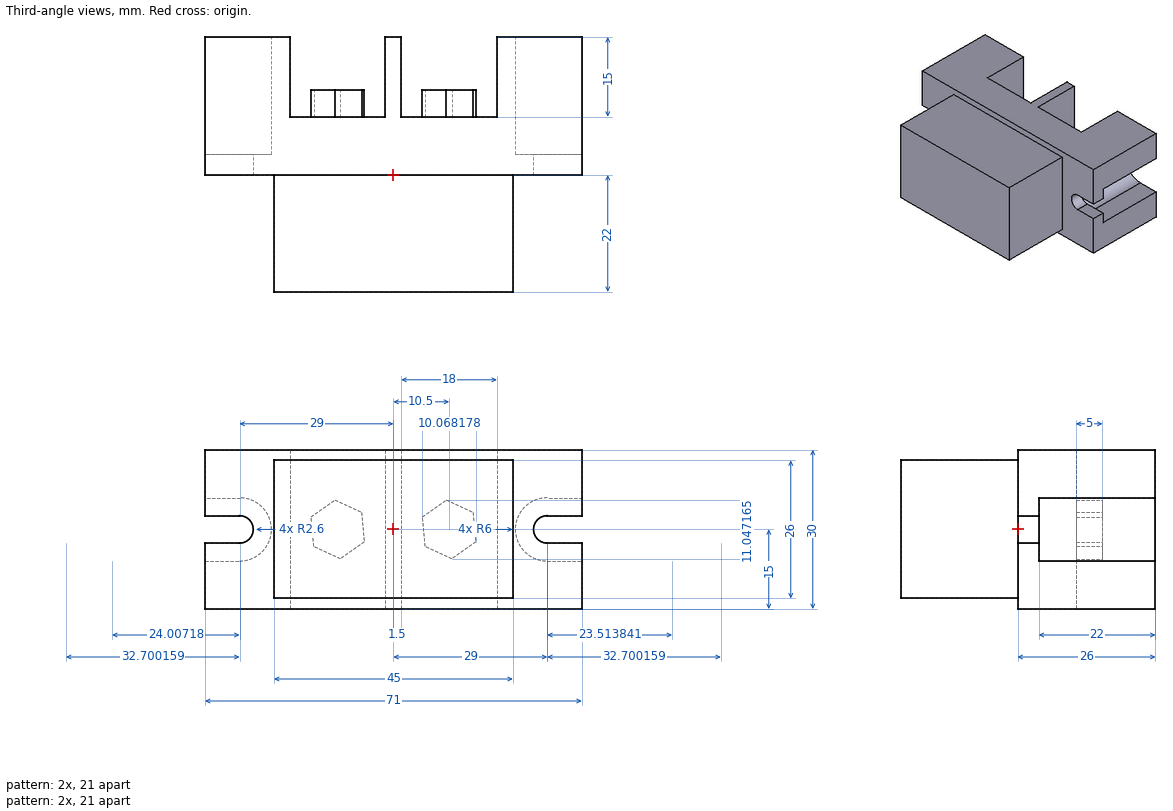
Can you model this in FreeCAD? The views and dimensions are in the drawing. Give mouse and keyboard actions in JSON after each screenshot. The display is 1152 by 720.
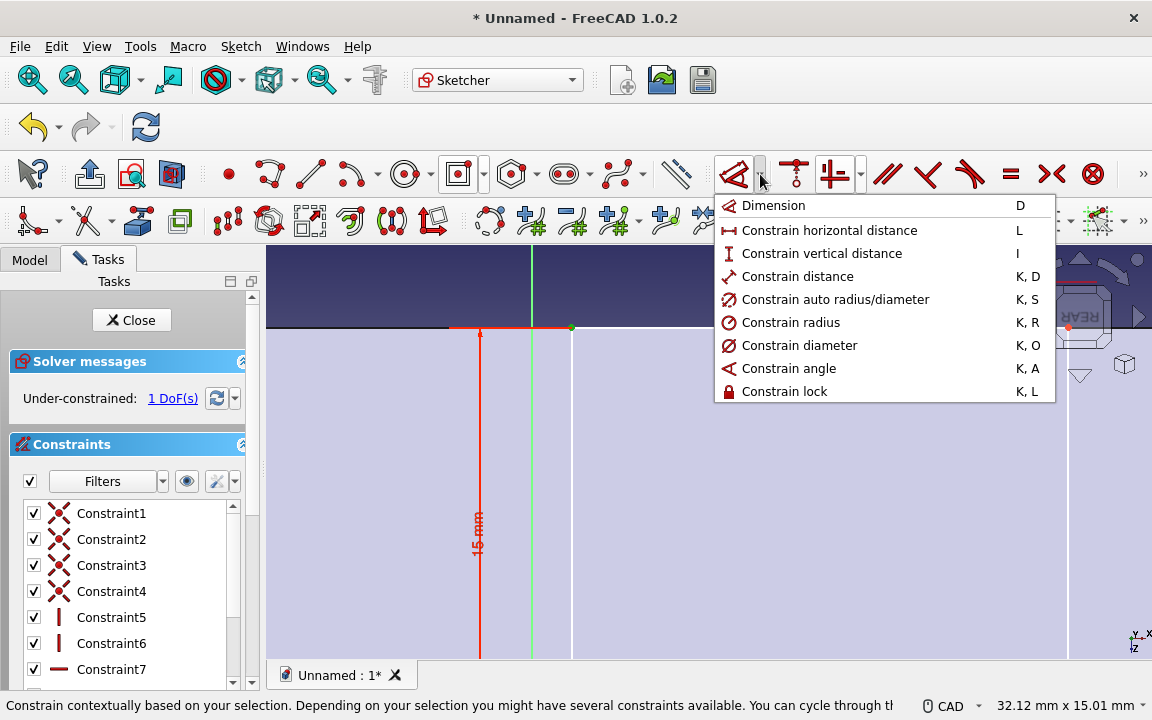
{"action": "left_click", "coordinate": [885, 230]}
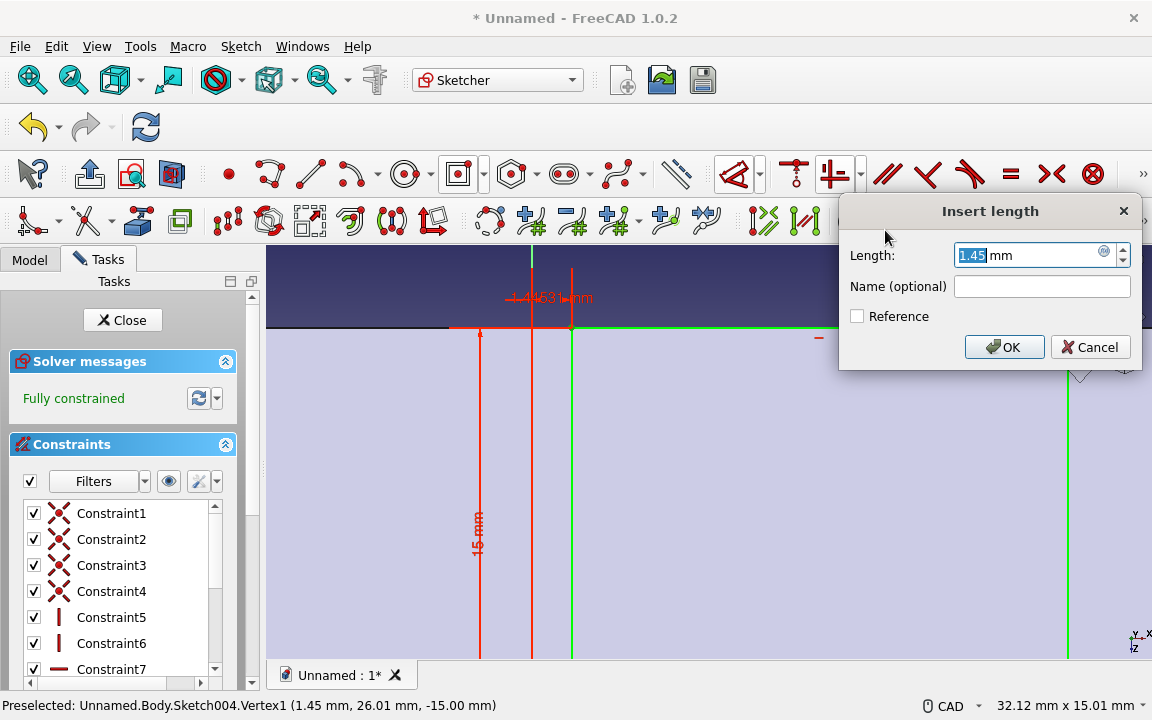
{"action": "type", "text": "1.5"}
{"action": "key", "text": "Return"}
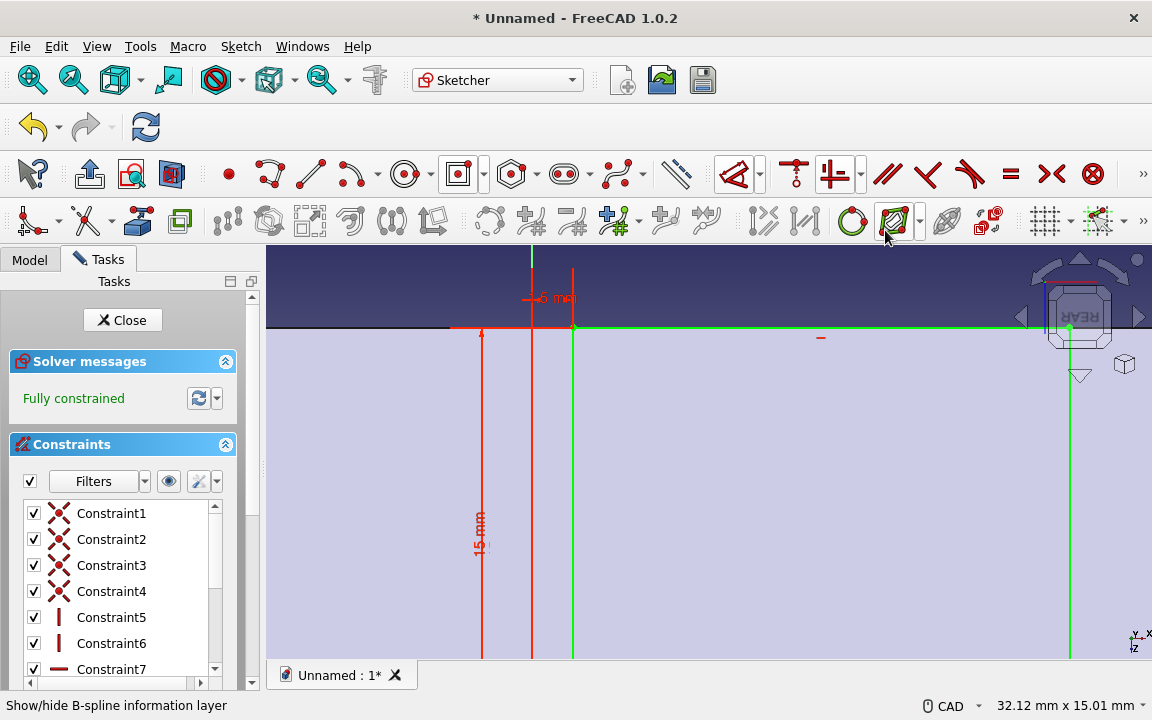
{"action": "left_click", "coordinate": [123, 320]}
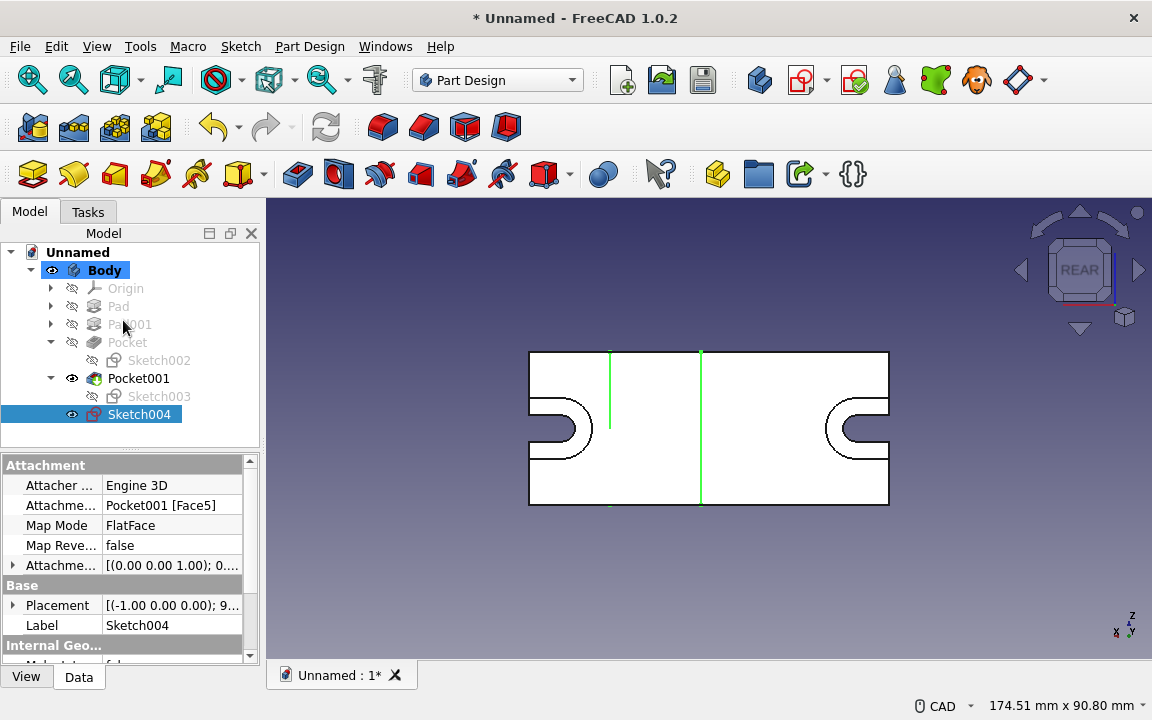
{"action": "left_click", "coordinate": [298, 174]}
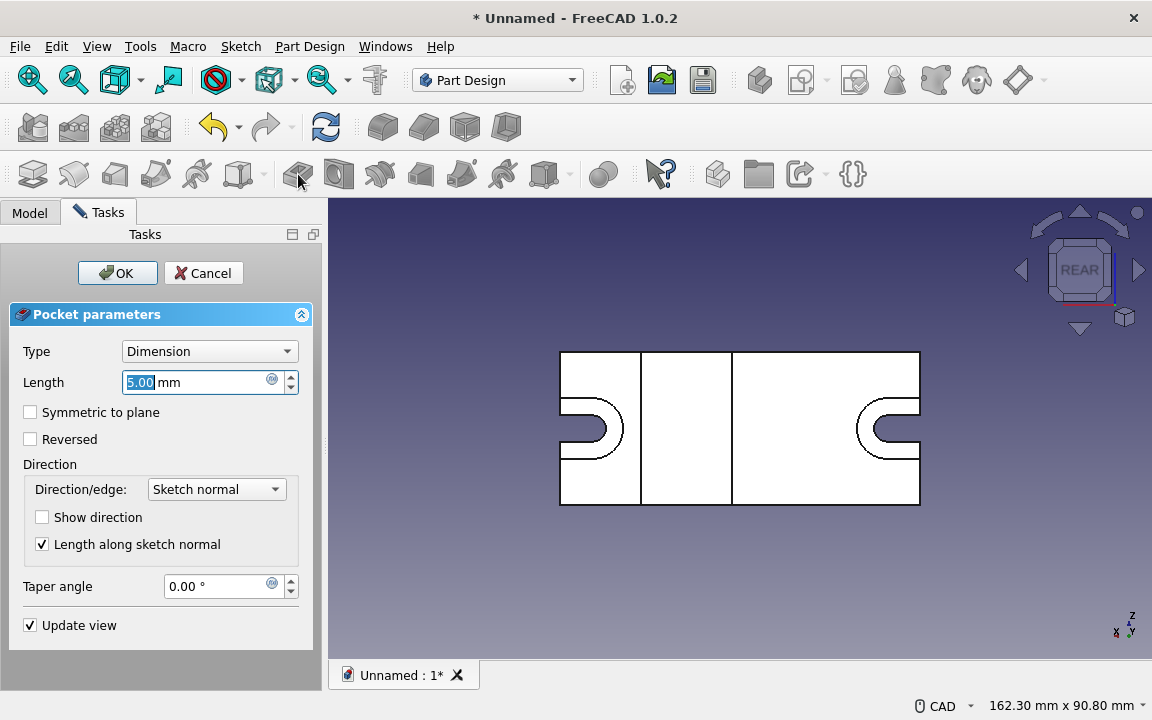
{"action": "type", "text": "15"}
{"action": "key", "text": "Tab"}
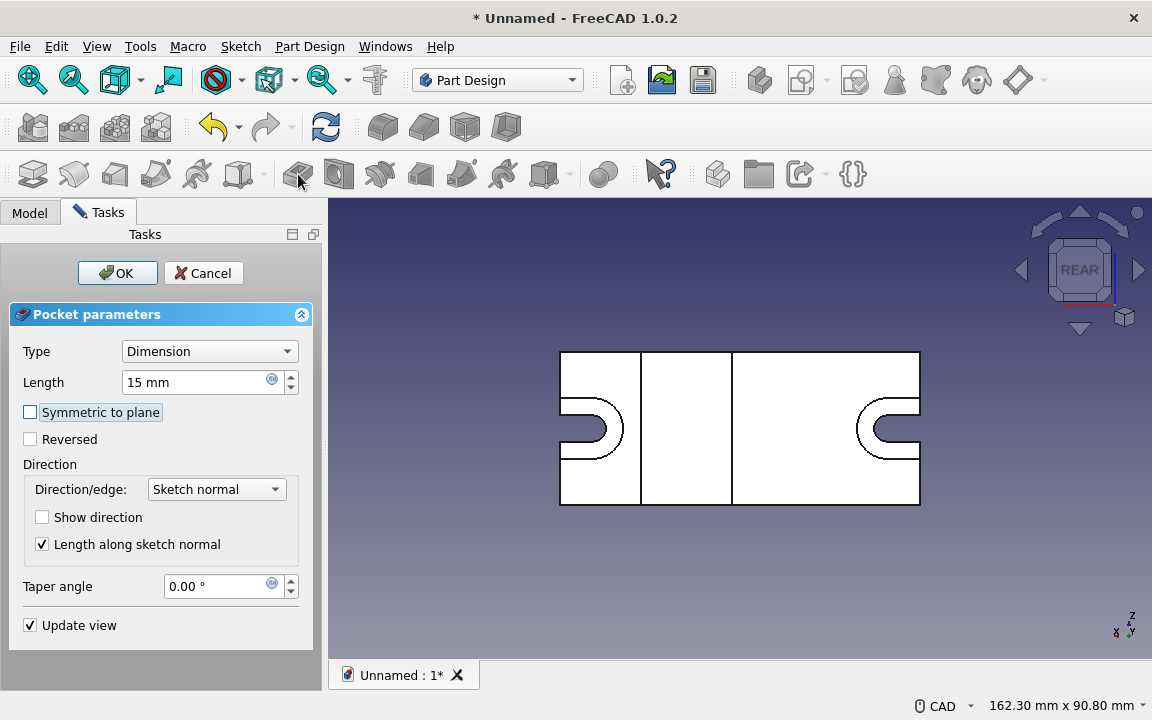
{"action": "left_click", "coordinate": [118, 273]}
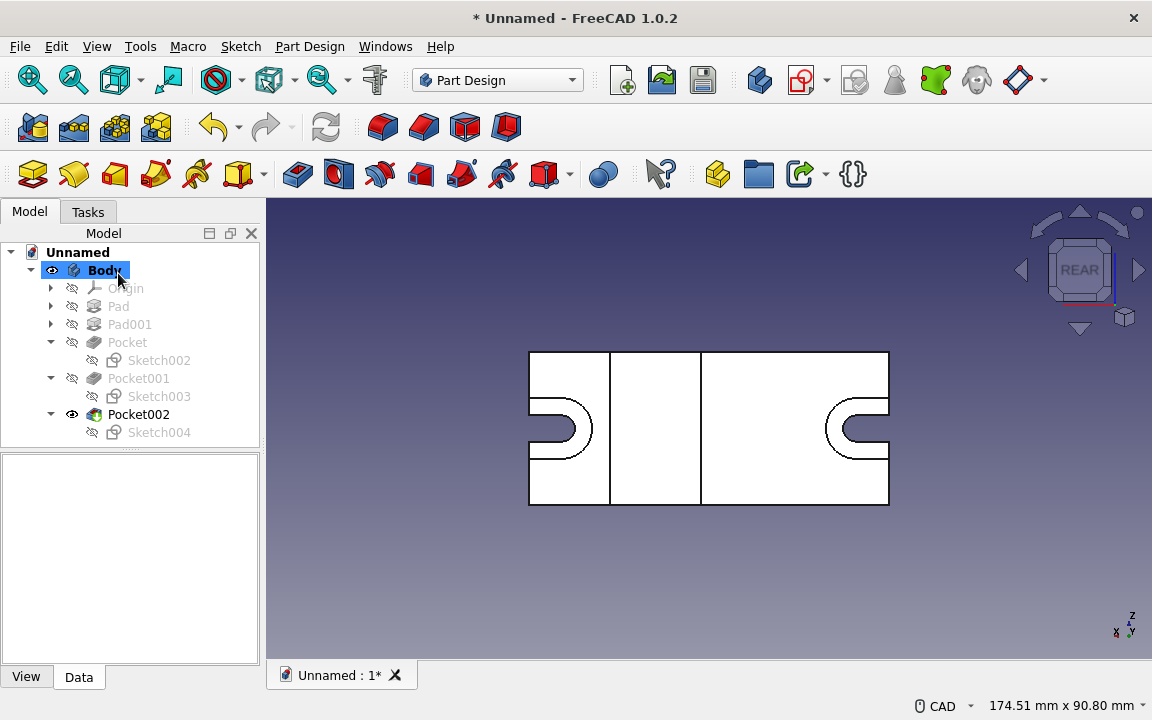
{"action": "left_click", "coordinate": [33, 80]}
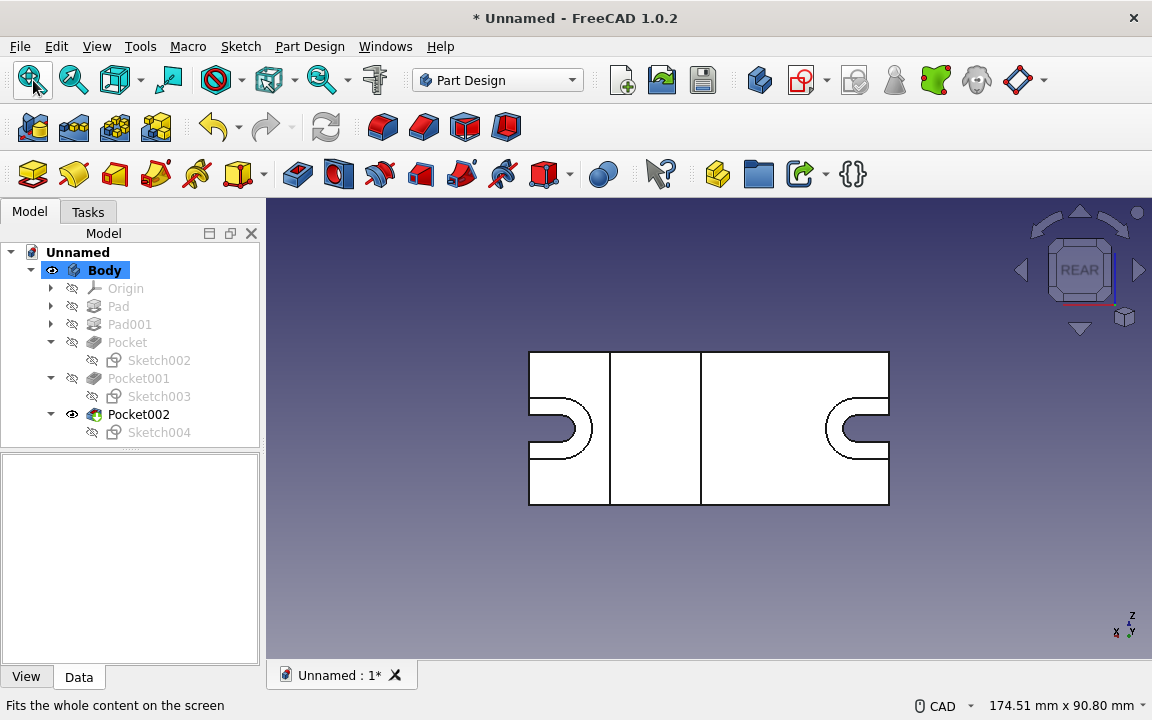
{"action": "left_click", "coordinate": [117, 414]}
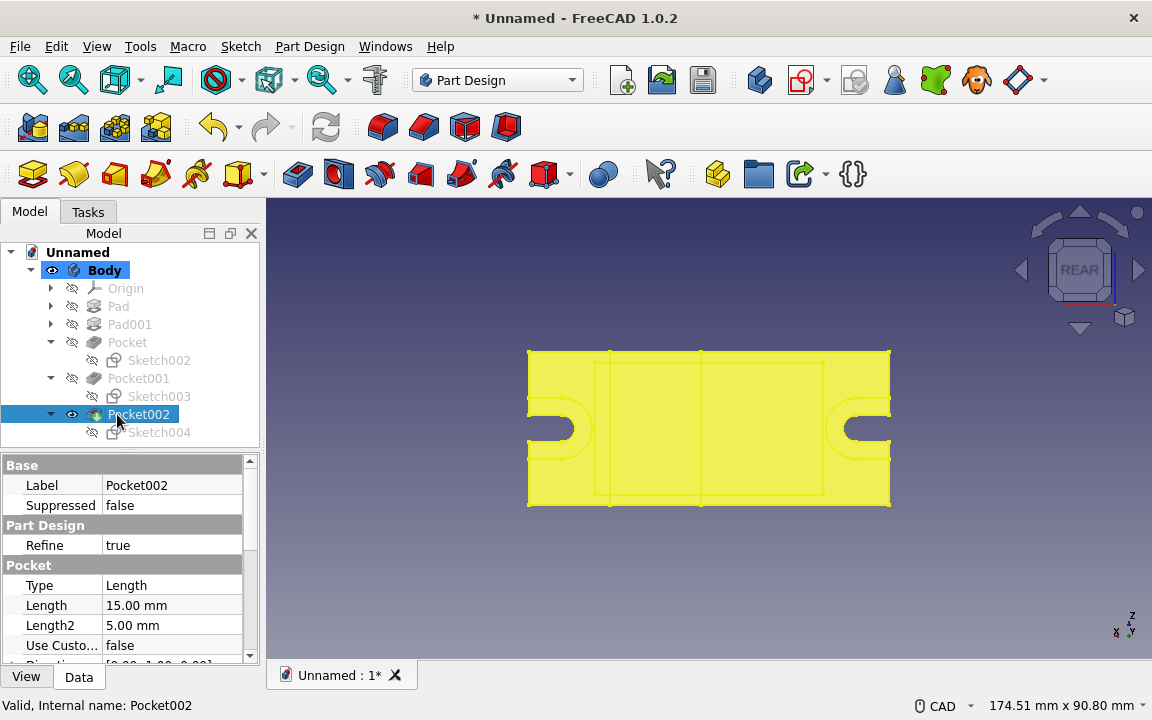
{"action": "left_click", "coordinate": [74, 128]}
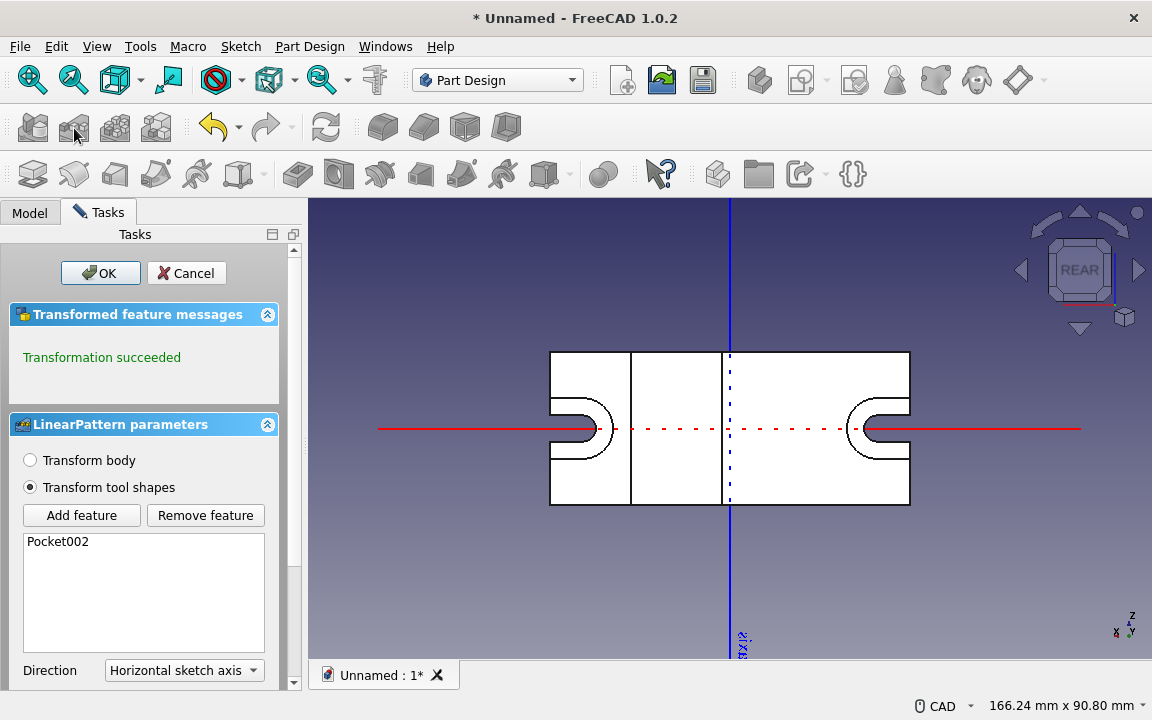
{"action": "left_click", "coordinate": [185, 670]}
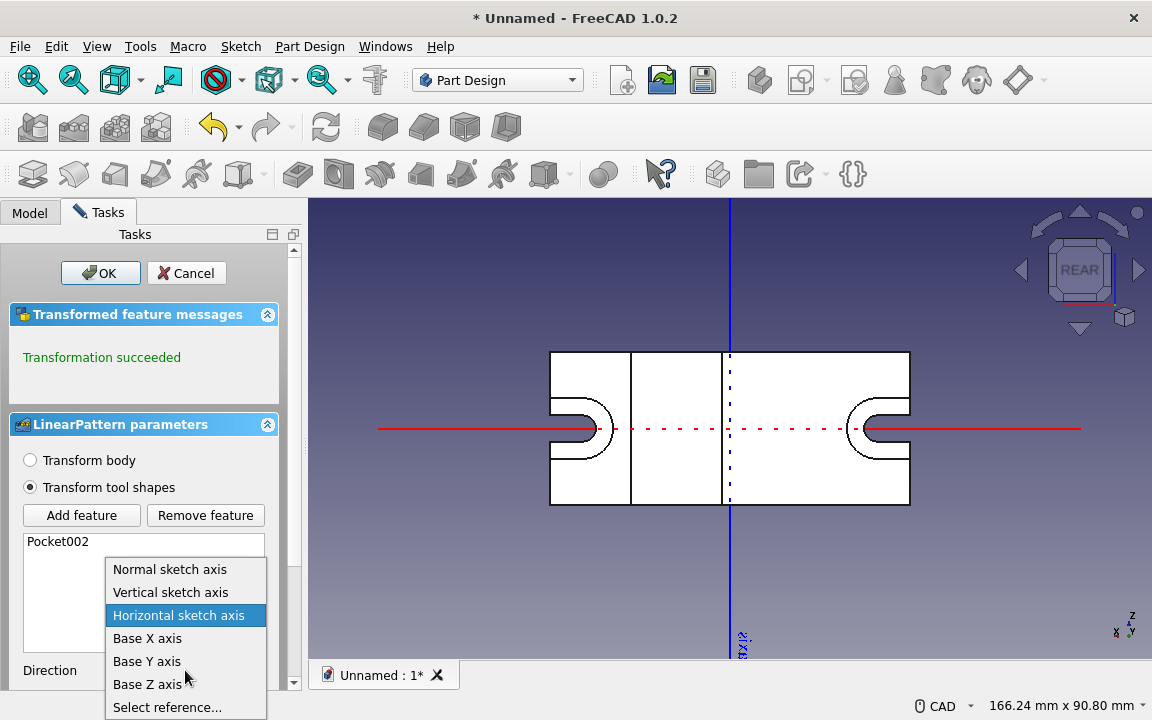
{"action": "left_click", "coordinate": [184, 638]}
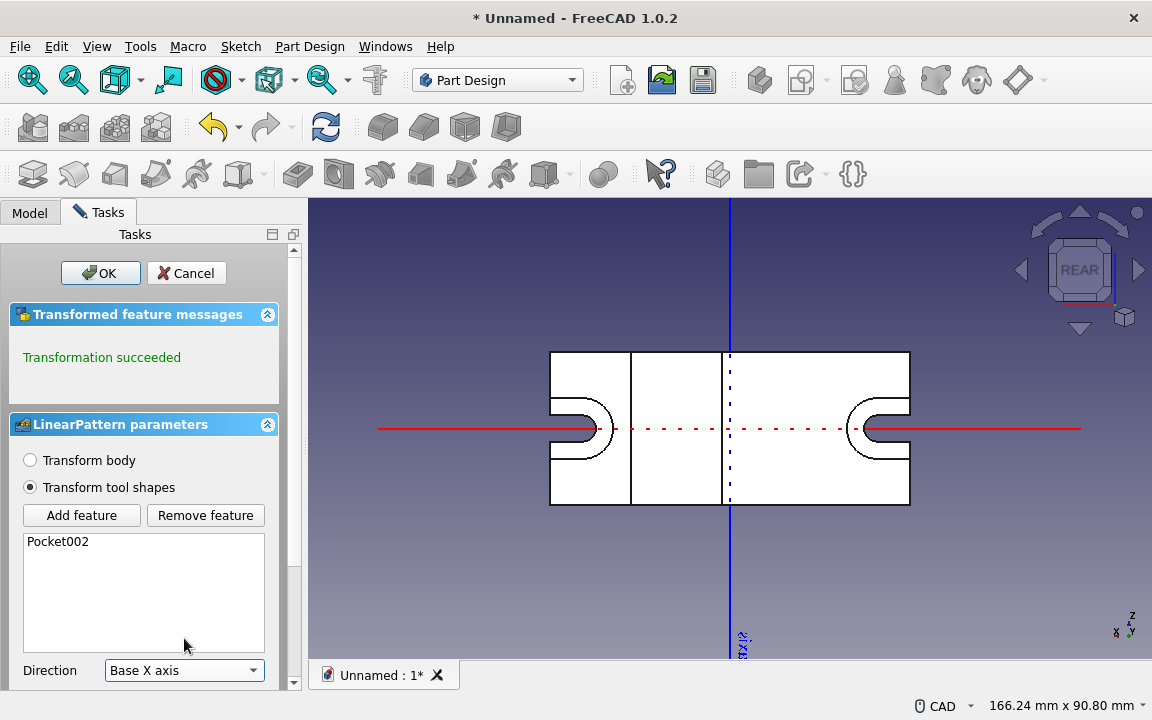
{"action": "scroll", "coordinate": [294, 467], "scroll_direction": "down", "scroll_amount": 2}